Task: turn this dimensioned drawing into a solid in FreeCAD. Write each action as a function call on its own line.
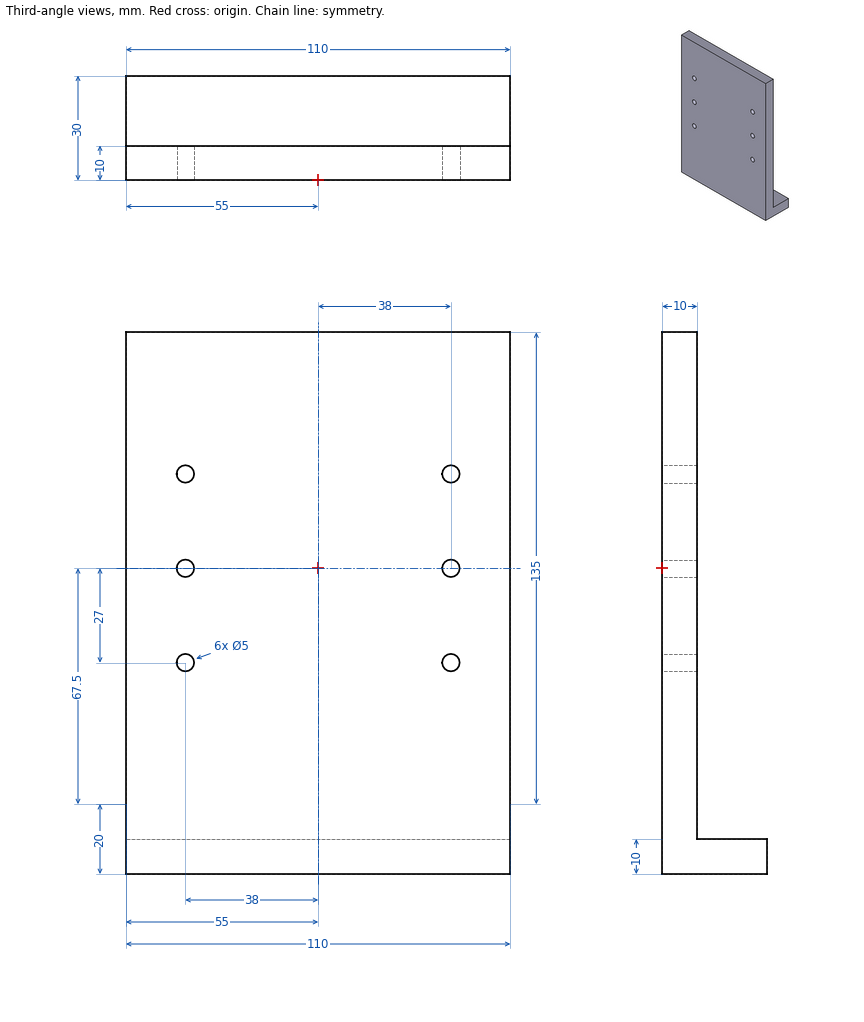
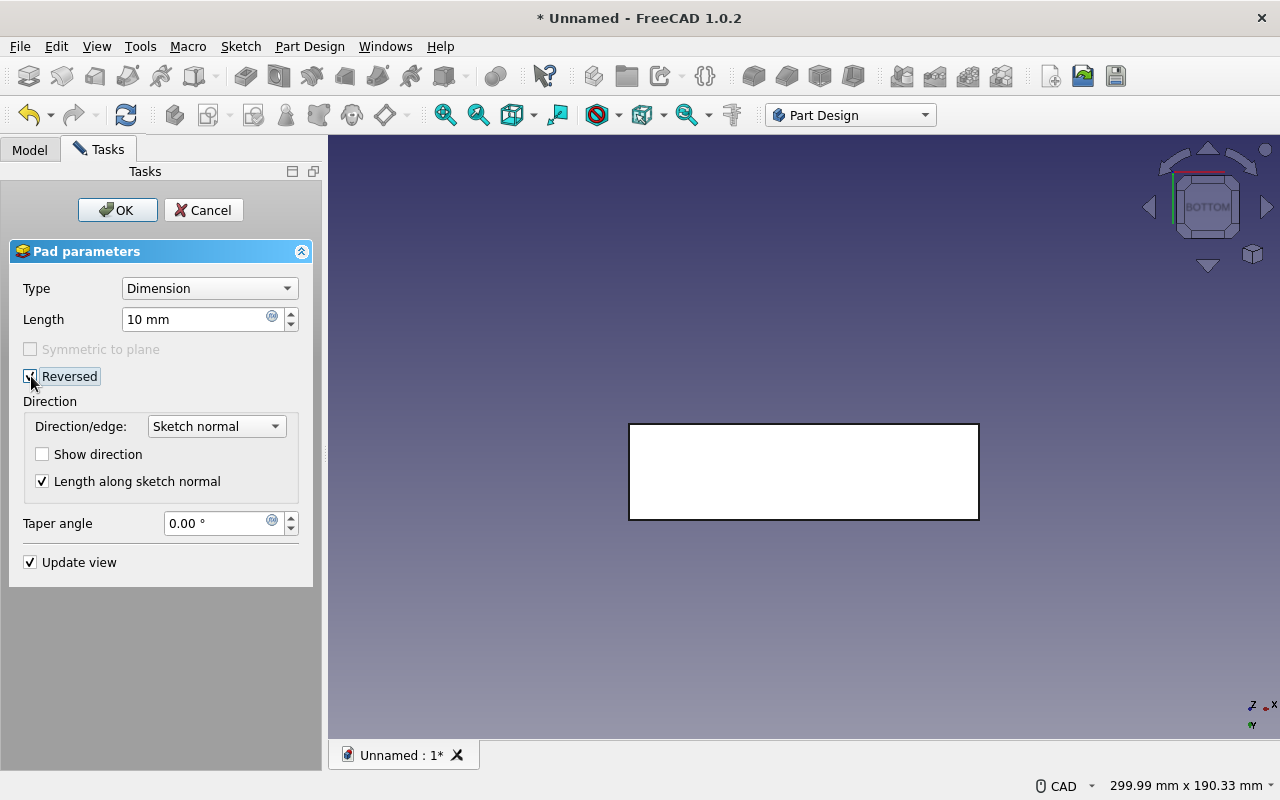
click(118, 210)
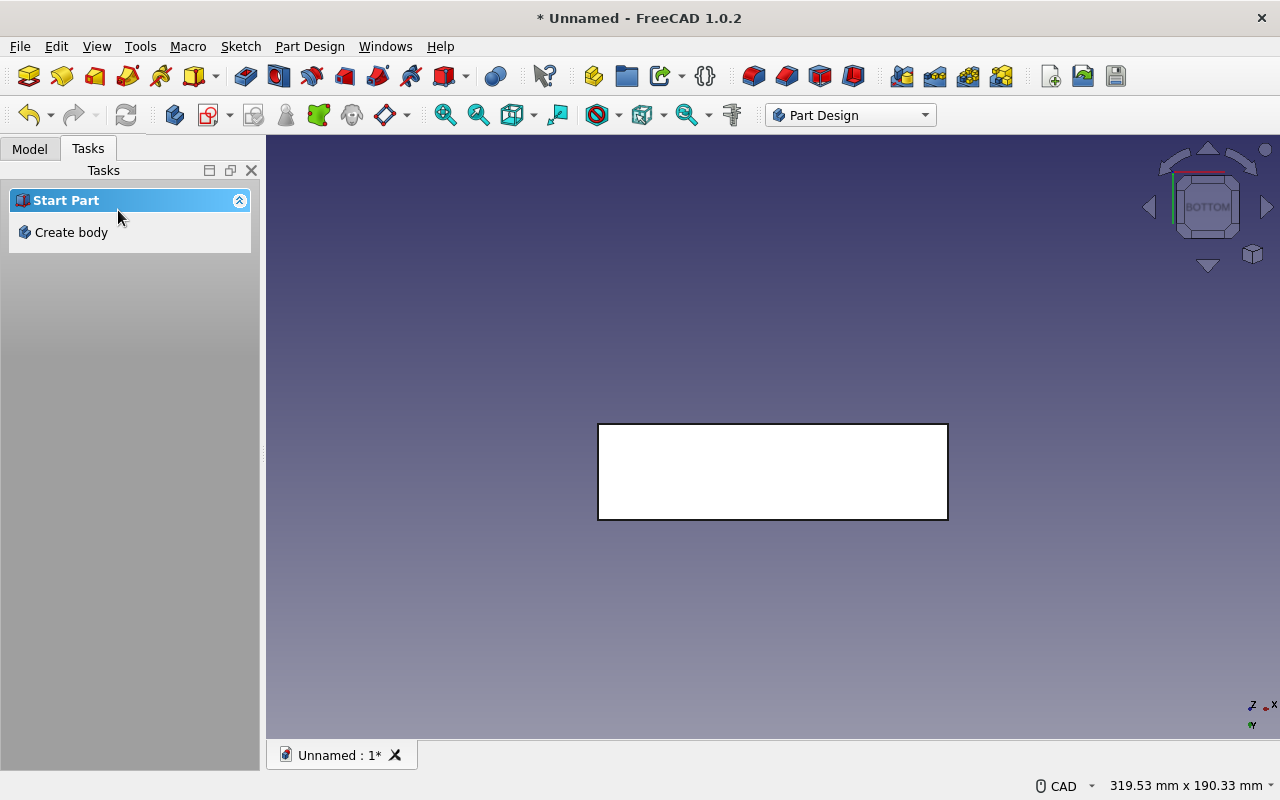
key(0)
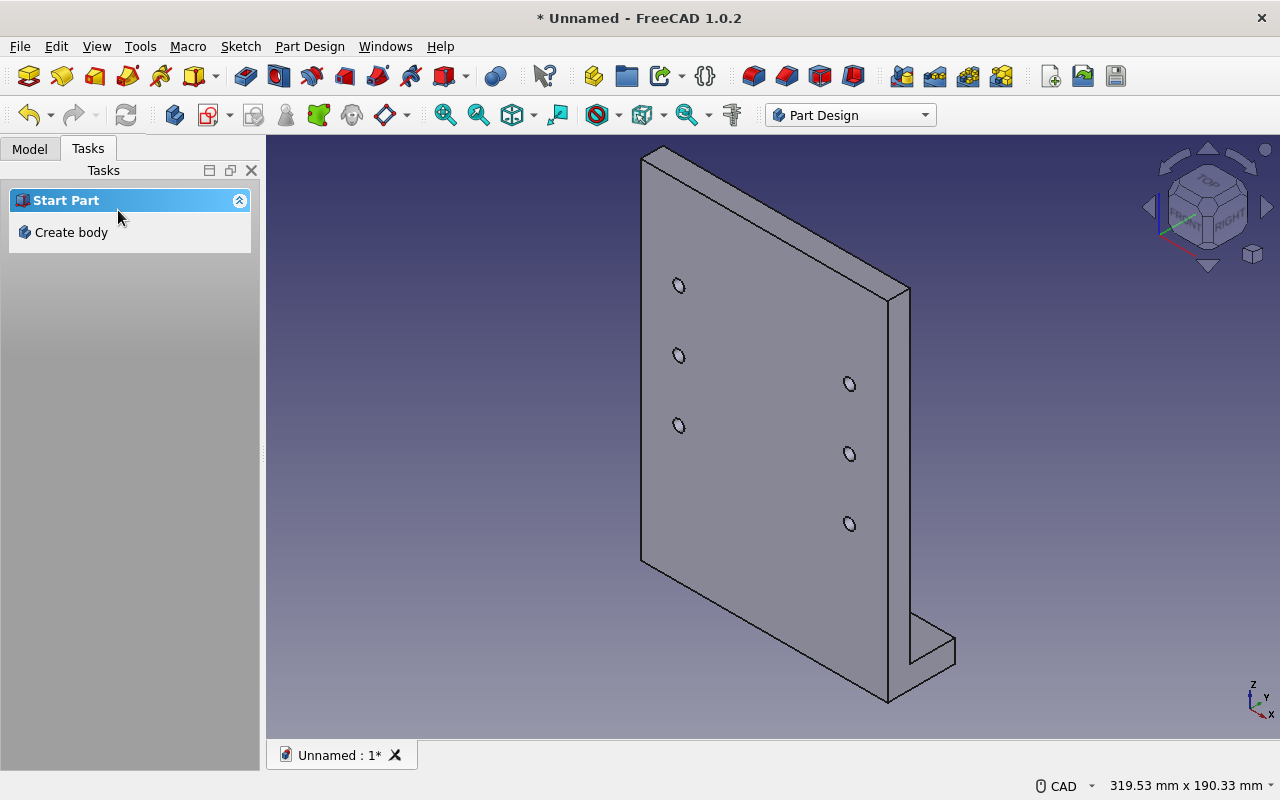
click(446, 116)